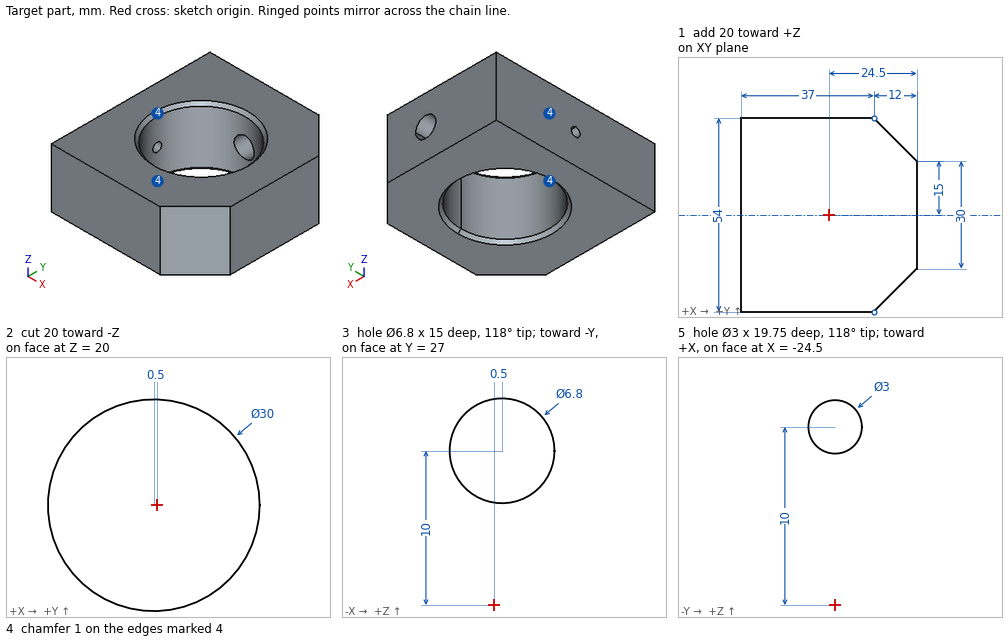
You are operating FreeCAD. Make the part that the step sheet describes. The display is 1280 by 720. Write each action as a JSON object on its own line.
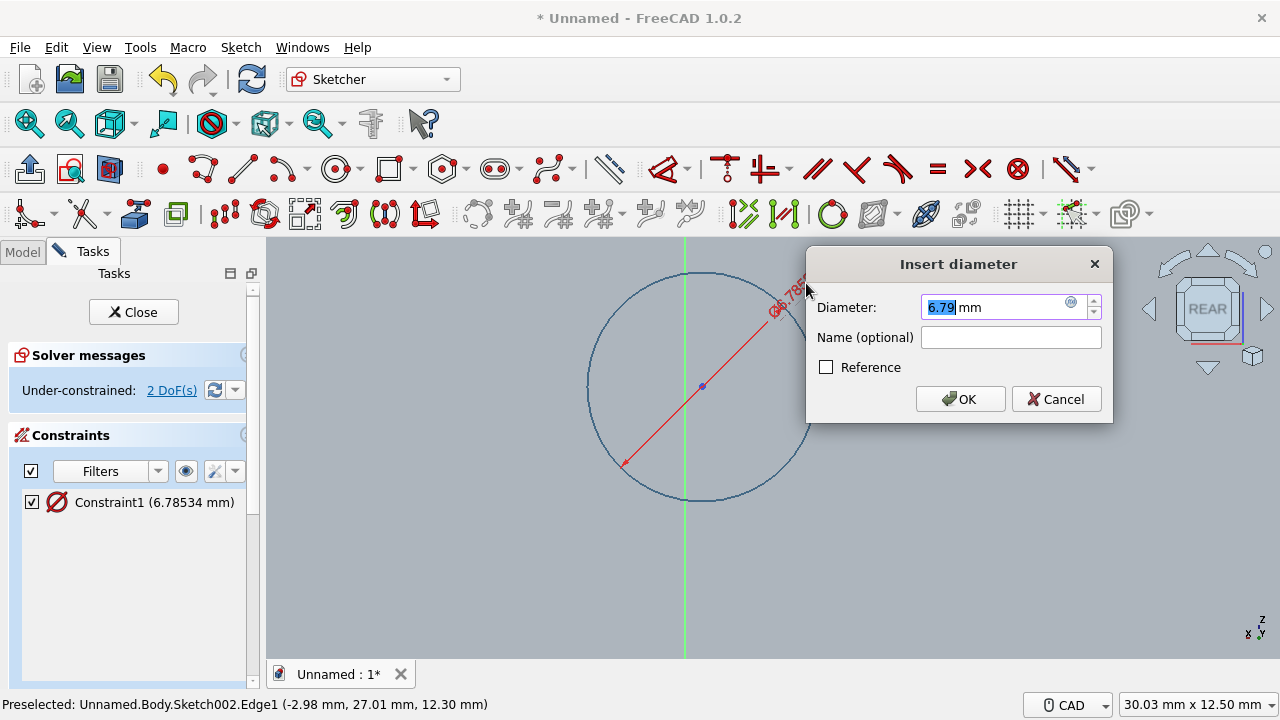
{"action": "type", "text": "6.8"}
{"action": "key", "text": "Return"}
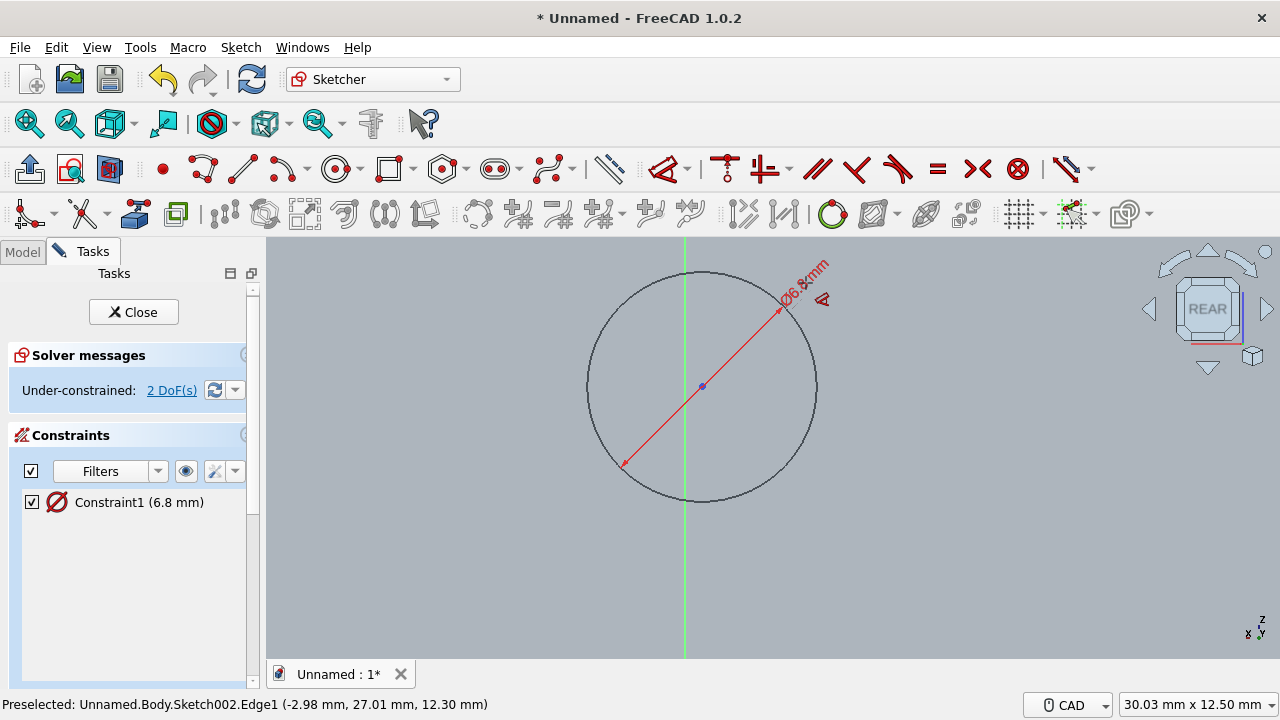
{"action": "left_click", "coordinate": [702, 387]}
{"action": "left_click", "coordinate": [651, 509]}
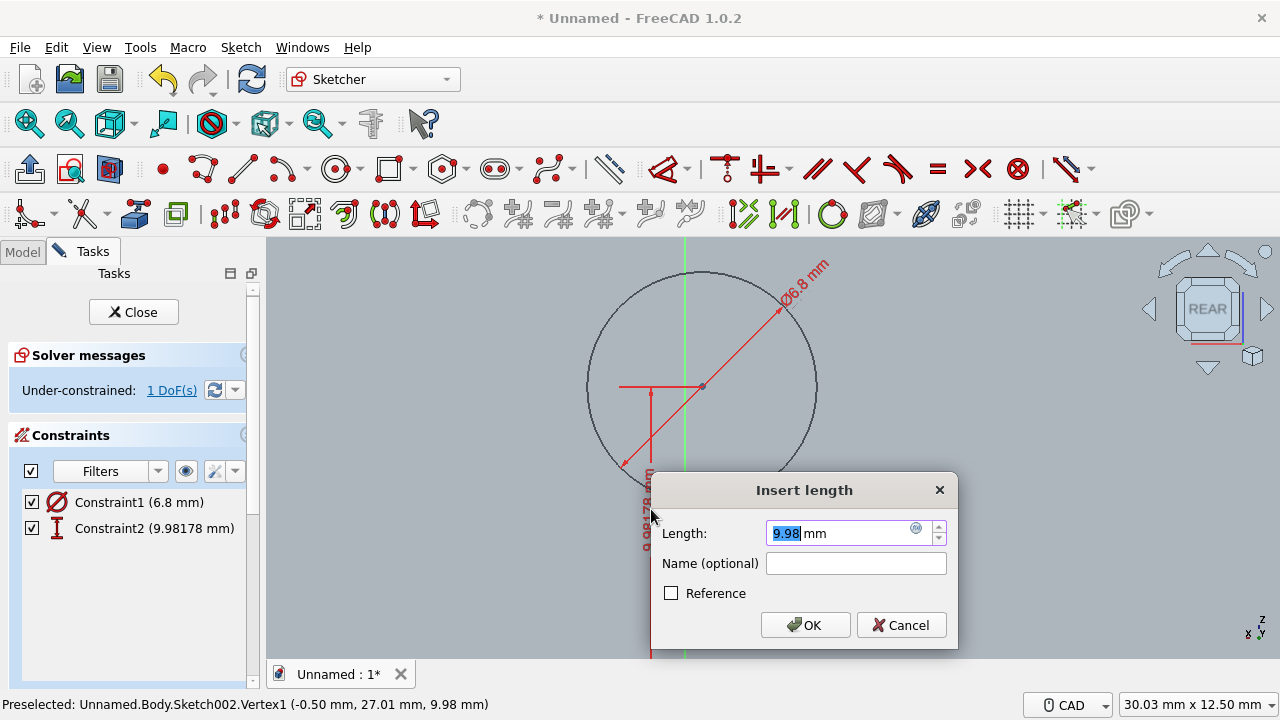
{"action": "type", "text": "10"}
{"action": "key", "text": "Return"}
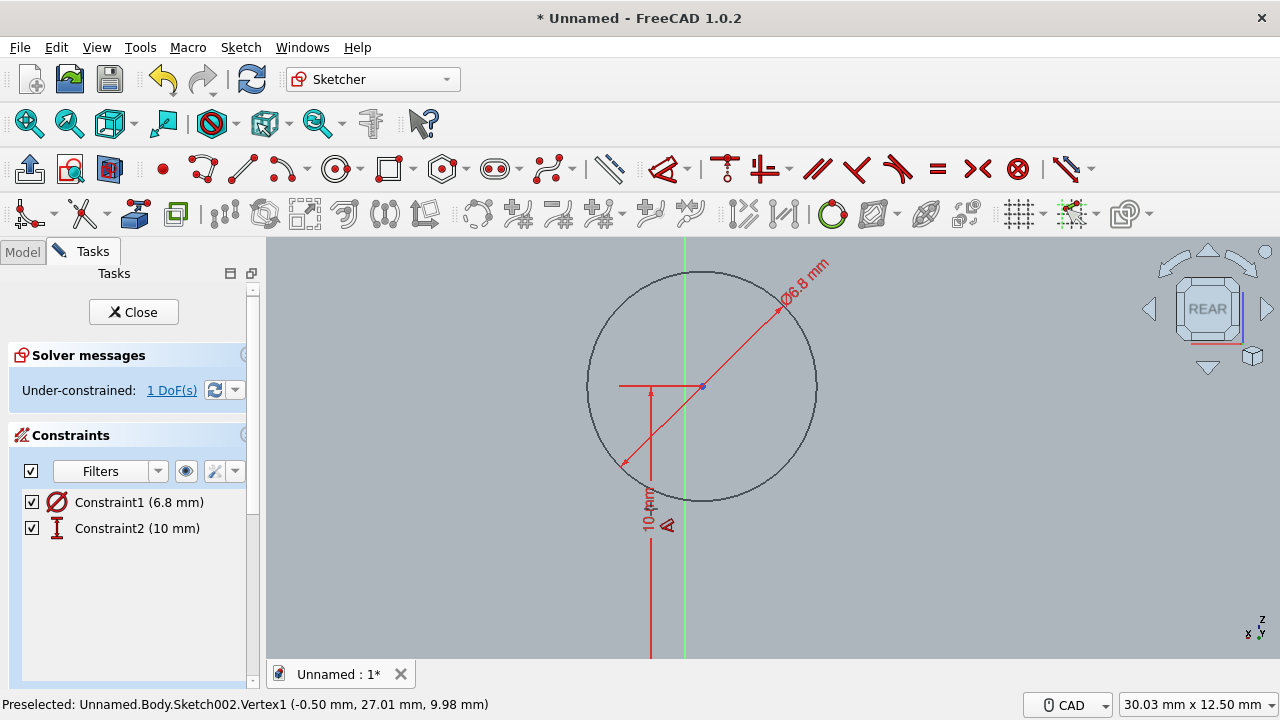
{"action": "scroll", "coordinate": [702, 386], "scroll_direction": "up", "scroll_amount": 5}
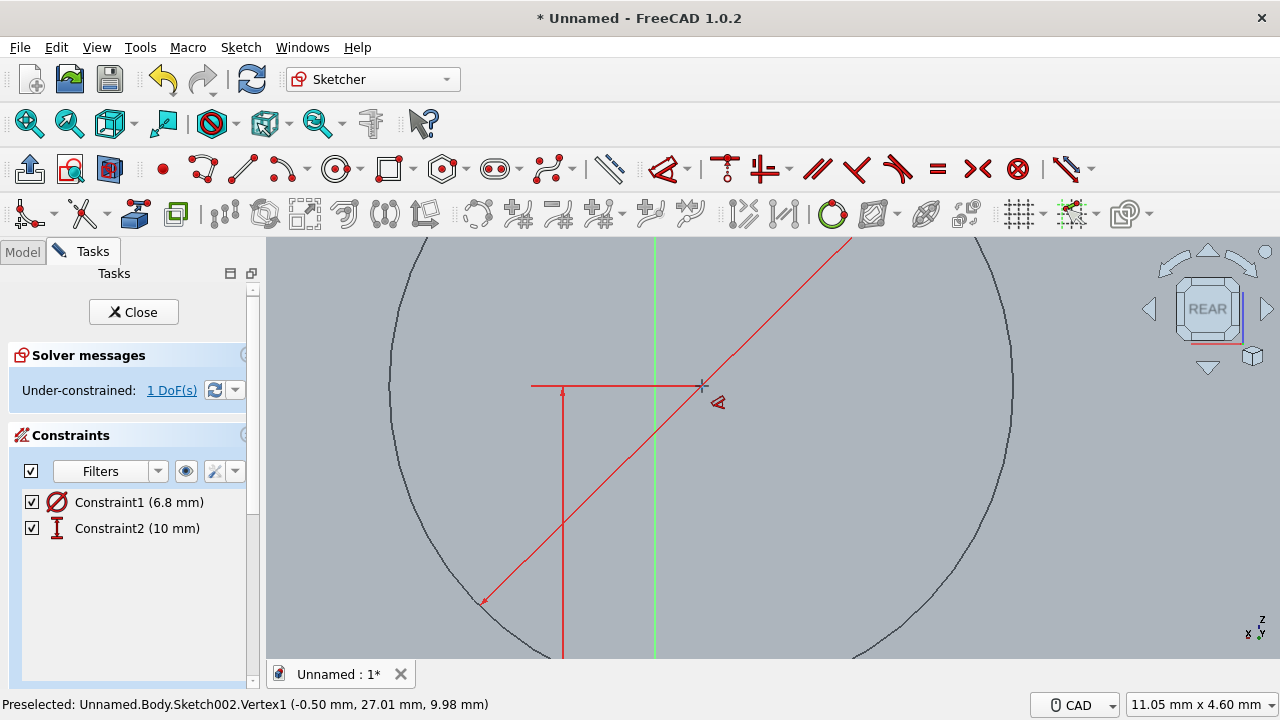
{"action": "left_click", "coordinate": [701, 386]}
{"action": "left_click", "coordinate": [678, 352]}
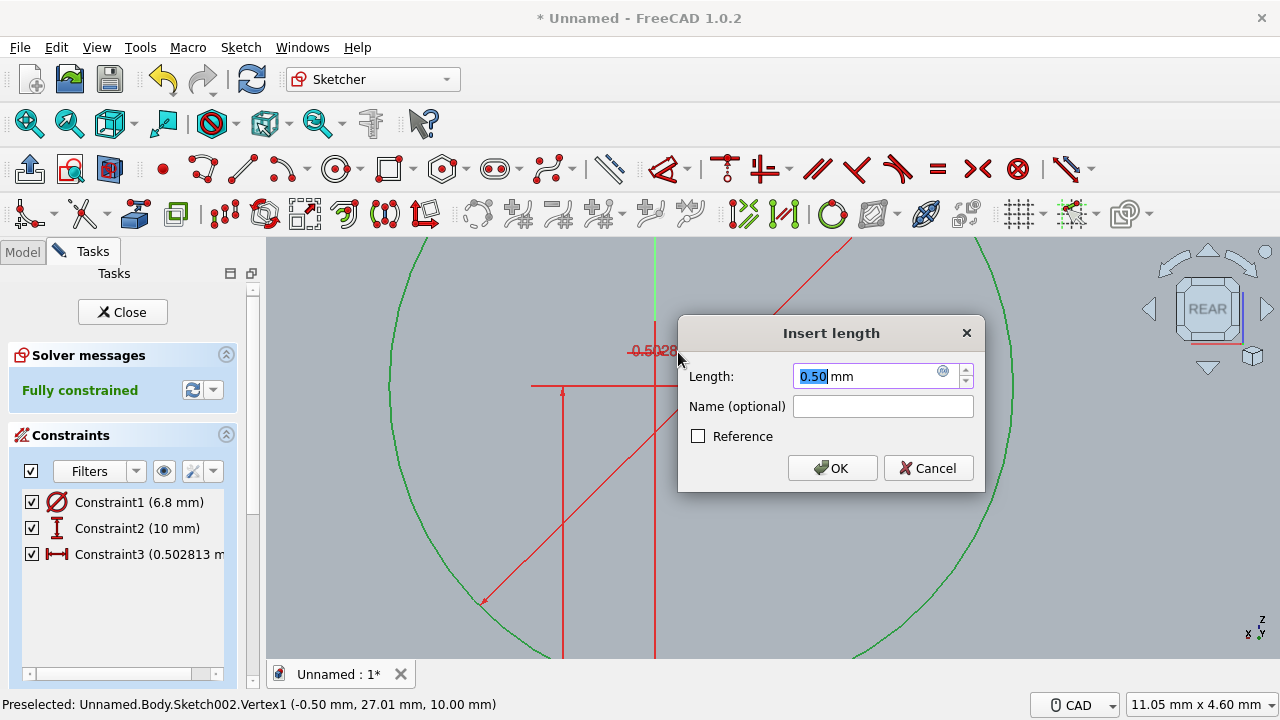
{"action": "type", "text": "0.5"}
{"action": "key", "text": "Return"}
{"action": "key", "text": "Escape"}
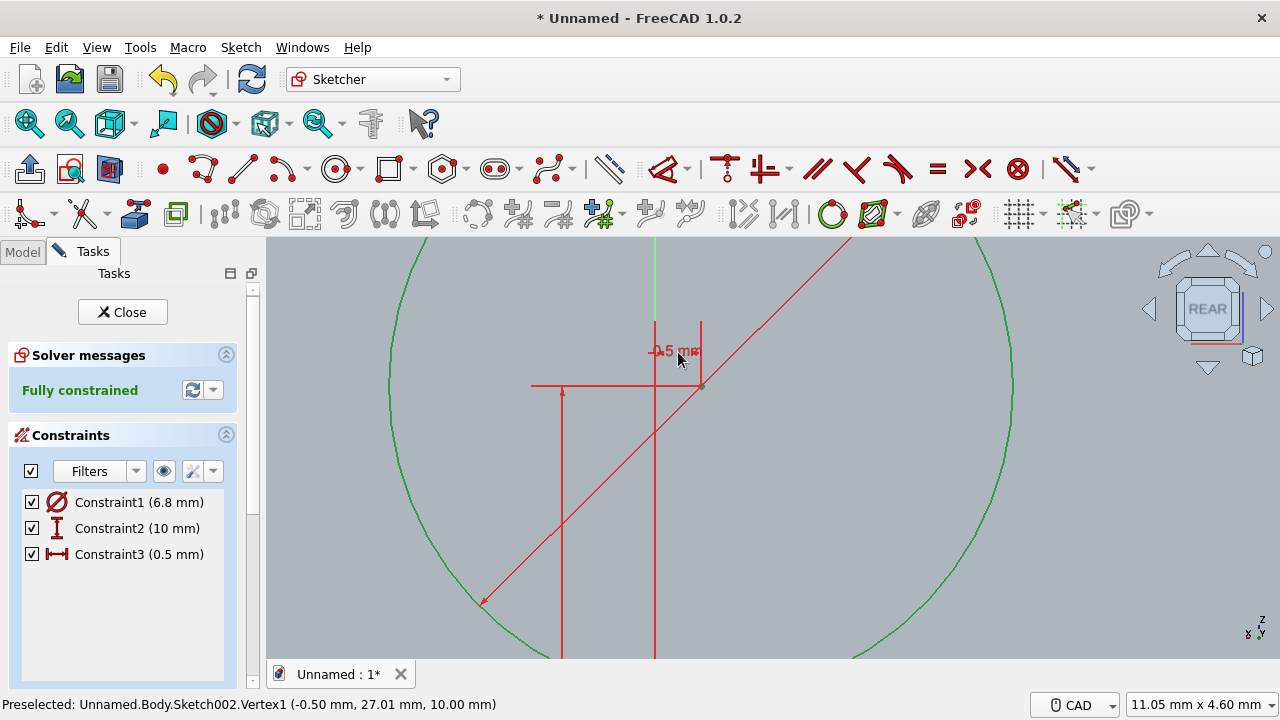
{"action": "left_click", "coordinate": [123, 312]}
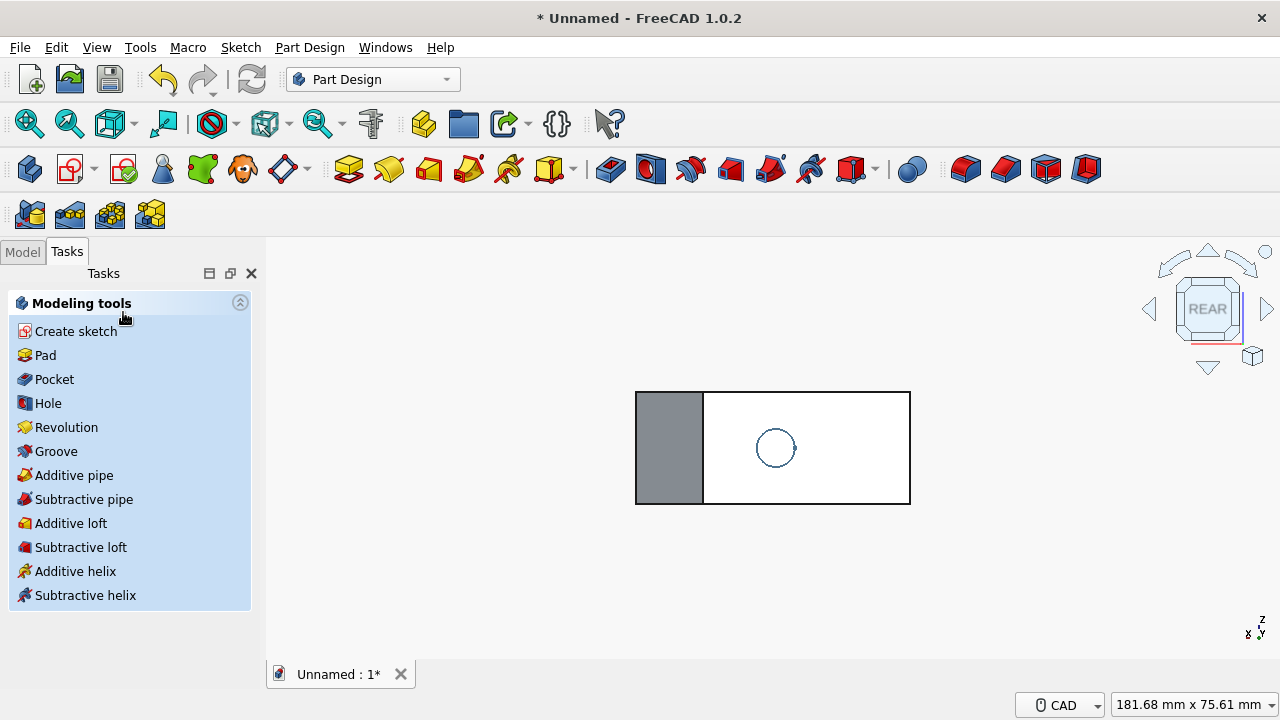
{"action": "left_click", "coordinate": [652, 170]}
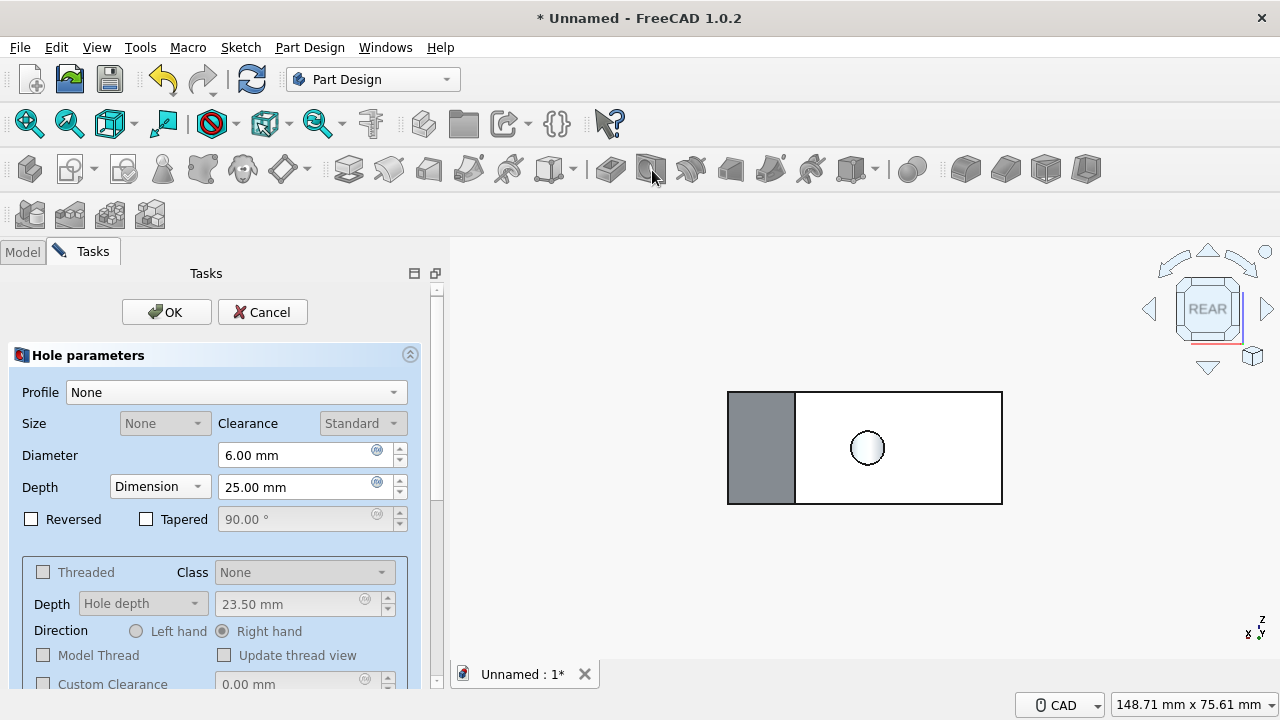
{"action": "triple_click", "coordinate": [305, 455]}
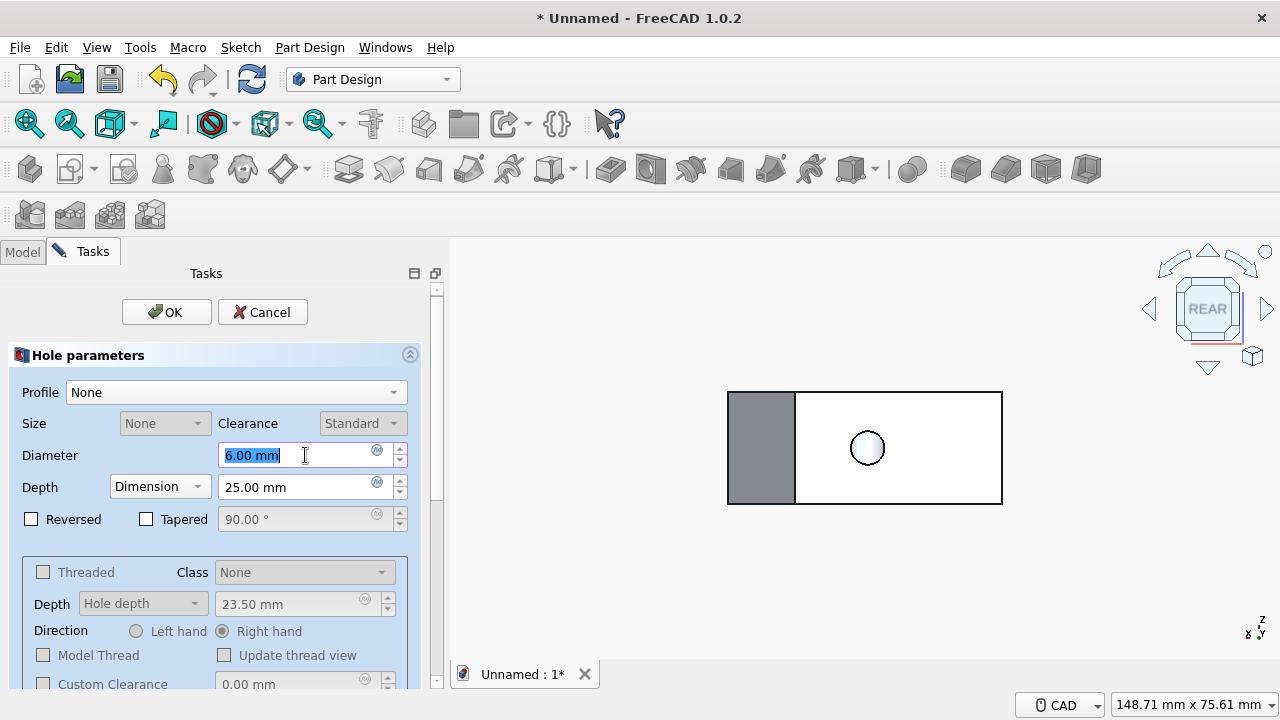
{"action": "type", "text": "6.8"}
{"action": "key", "text": "Tab"}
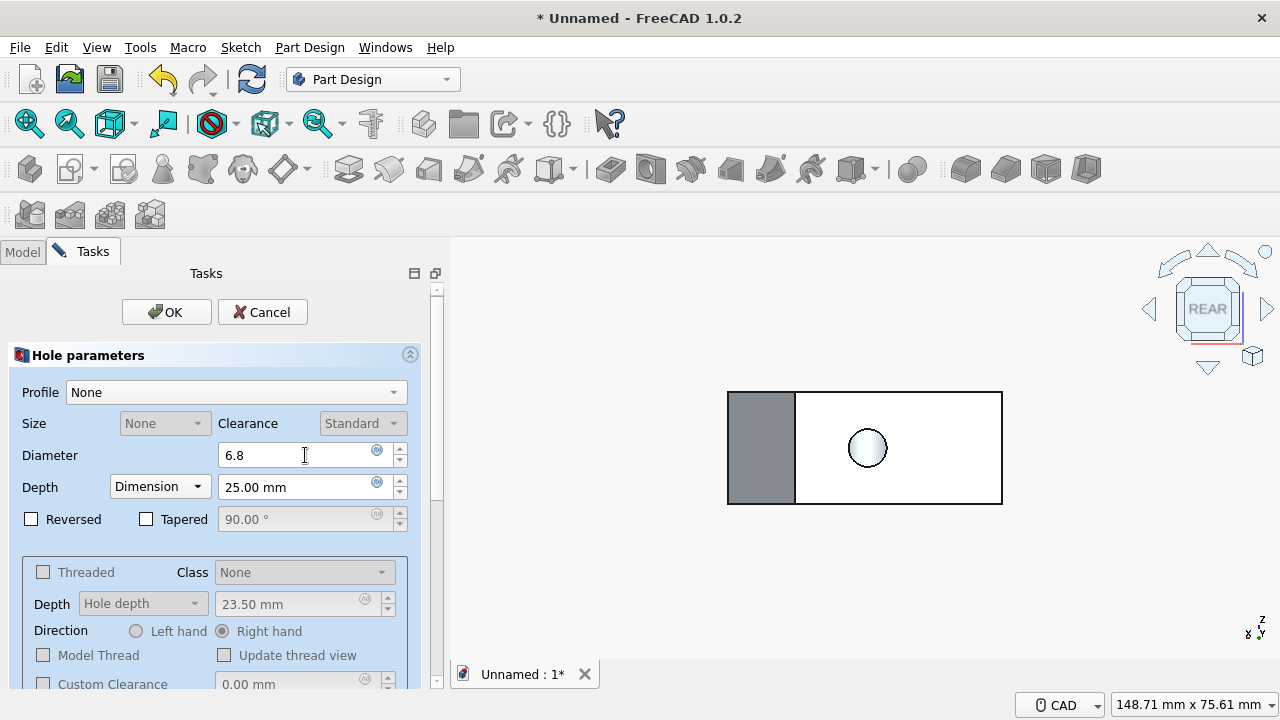
{"action": "triple_click", "coordinate": [305, 487]}